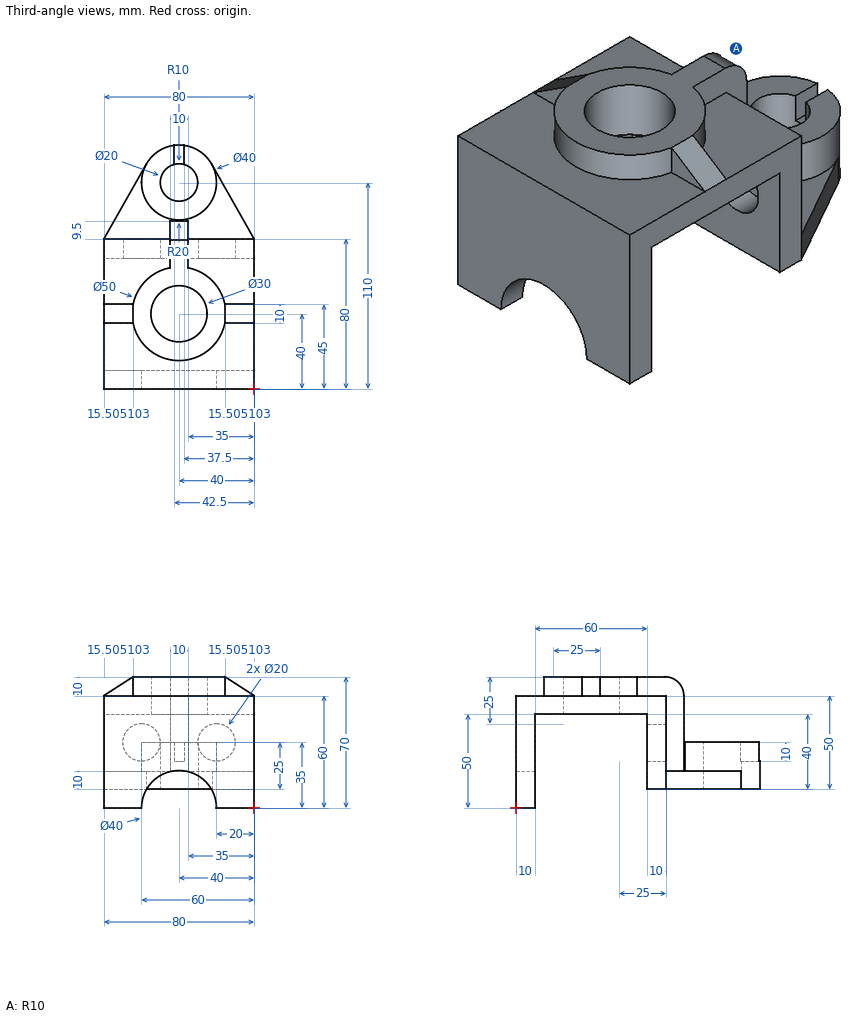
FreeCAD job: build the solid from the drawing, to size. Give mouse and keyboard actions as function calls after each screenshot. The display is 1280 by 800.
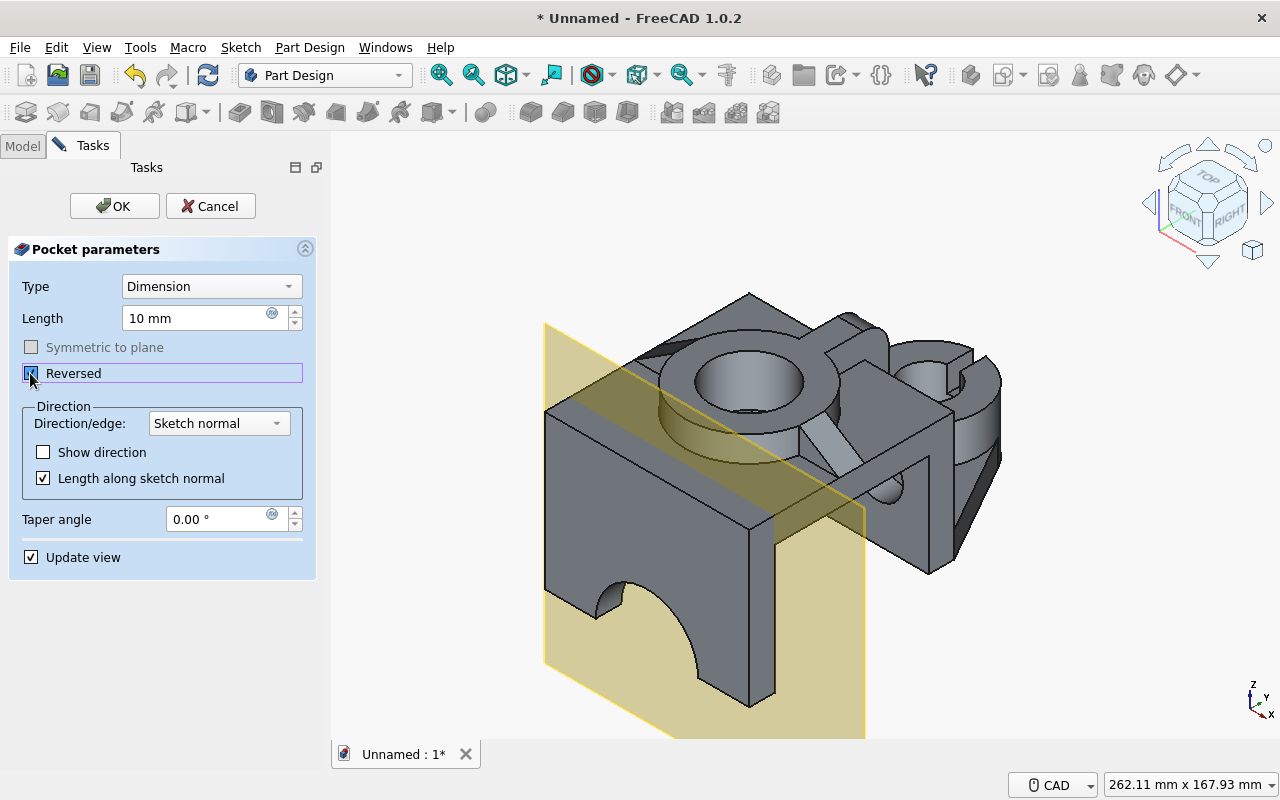
click(115, 206)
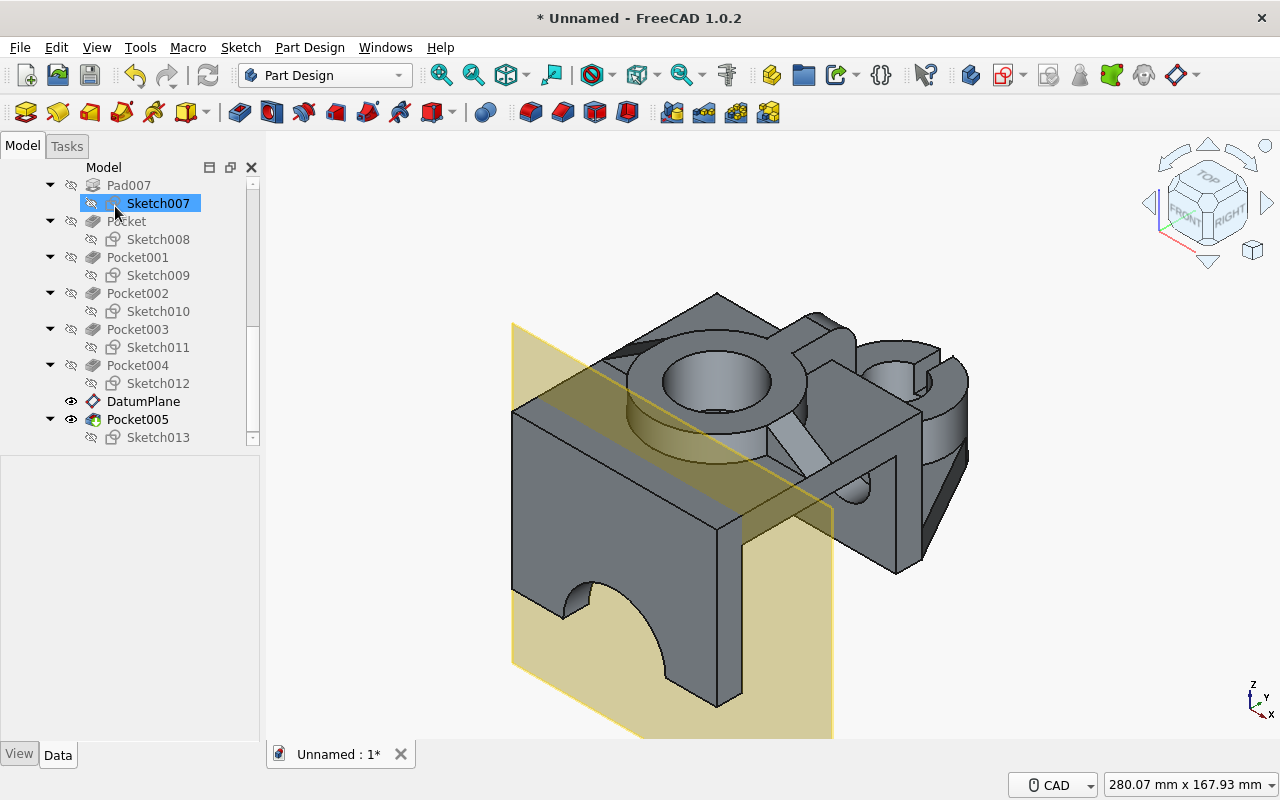
click(116, 401)
key(space)